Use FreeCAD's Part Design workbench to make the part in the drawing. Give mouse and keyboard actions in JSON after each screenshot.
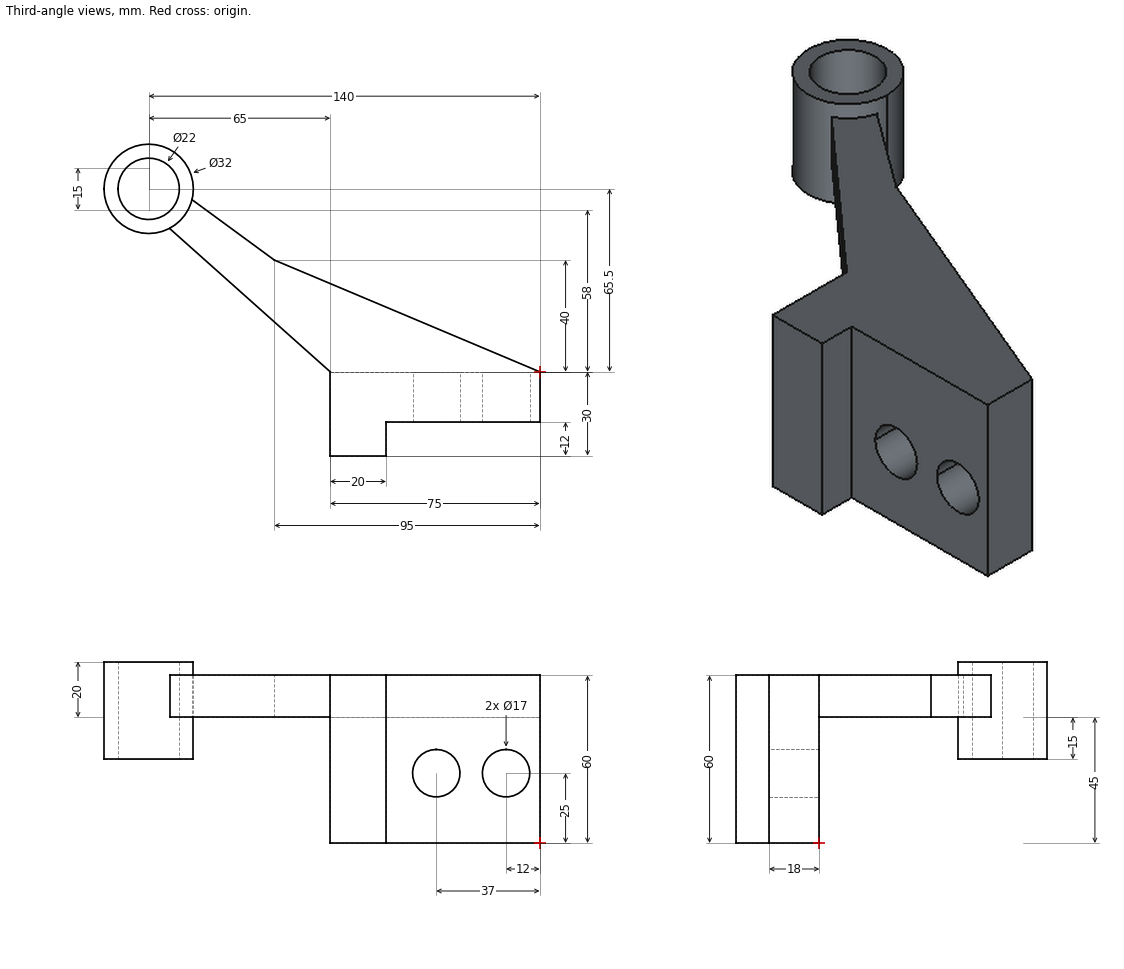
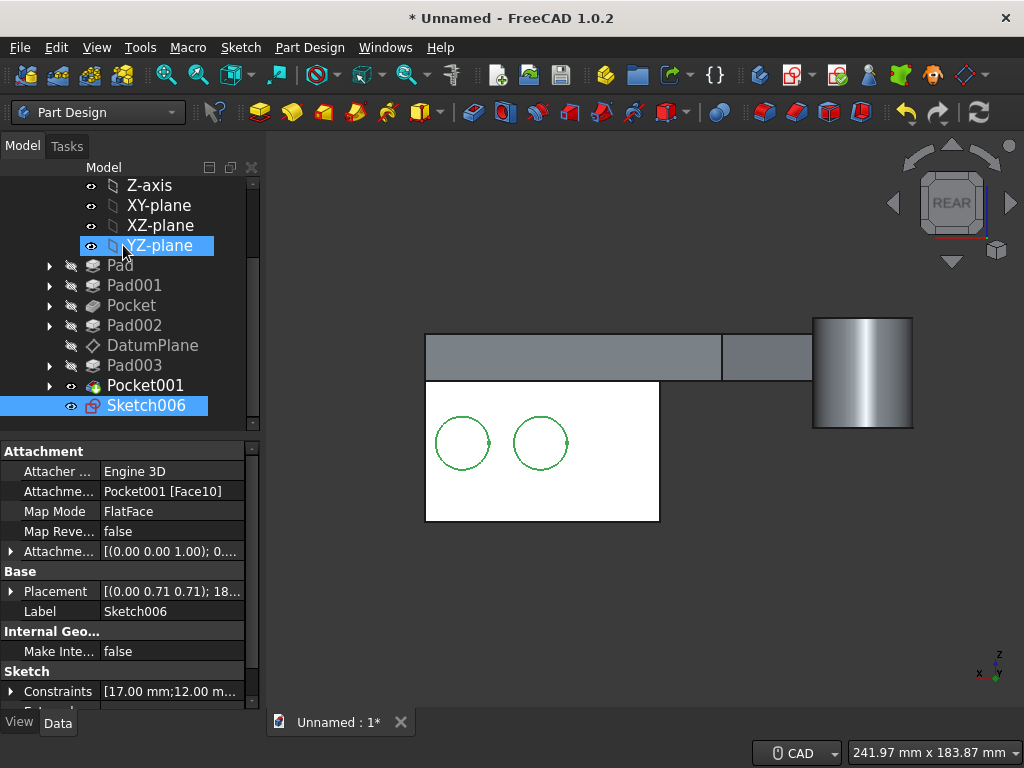
{"action": "left_click", "coordinate": [474, 112]}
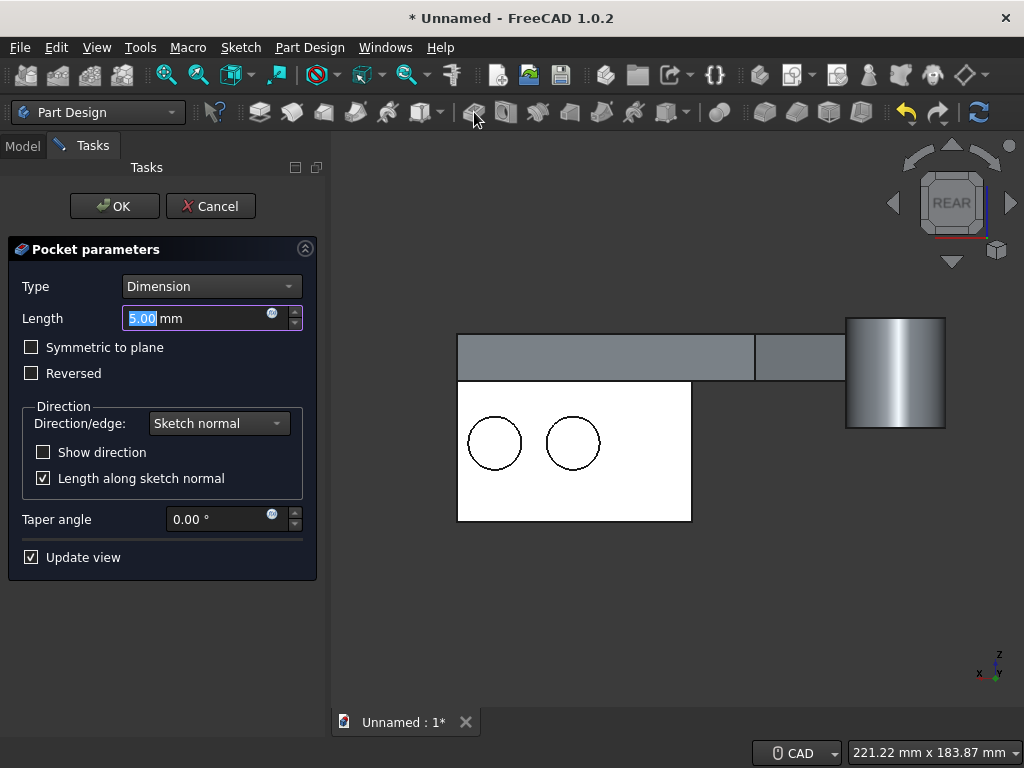
{"action": "type", "text": "18"}
{"action": "key", "text": "Tab"}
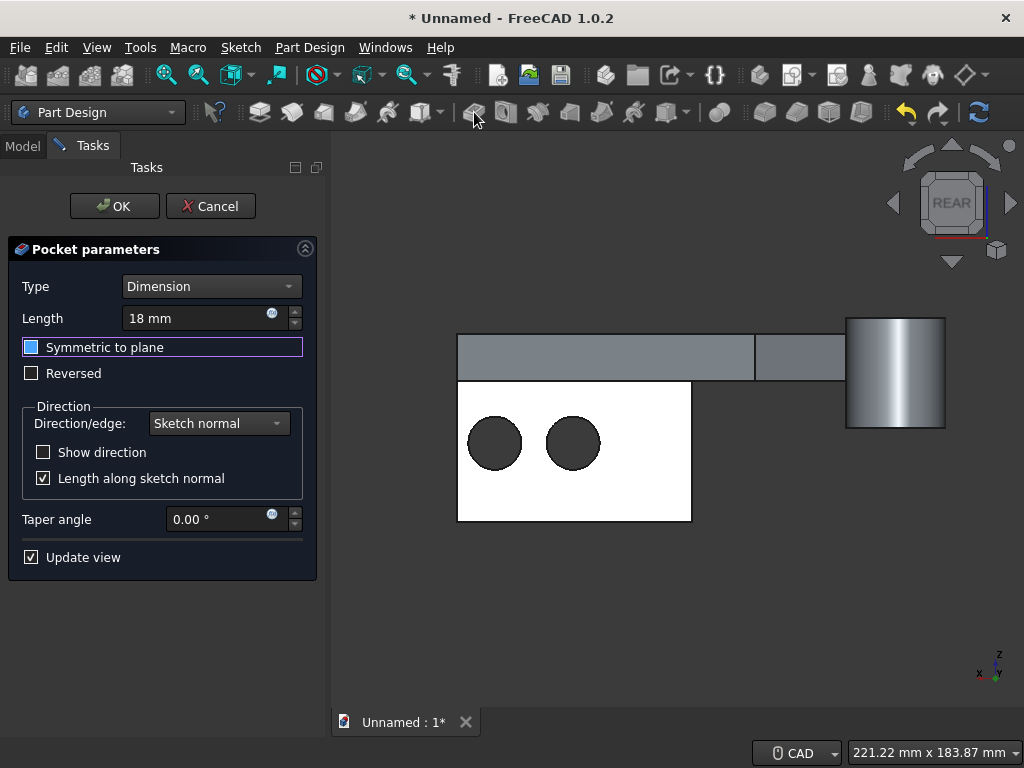
{"action": "left_click", "coordinate": [115, 206]}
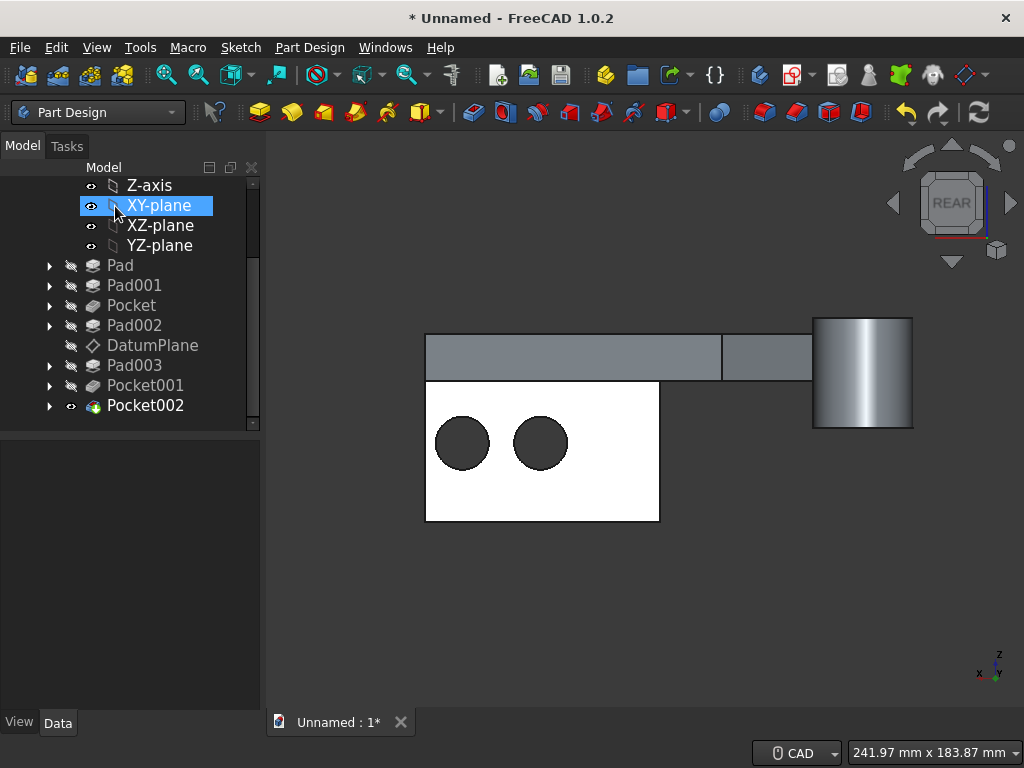
{"action": "key", "text": "0"}